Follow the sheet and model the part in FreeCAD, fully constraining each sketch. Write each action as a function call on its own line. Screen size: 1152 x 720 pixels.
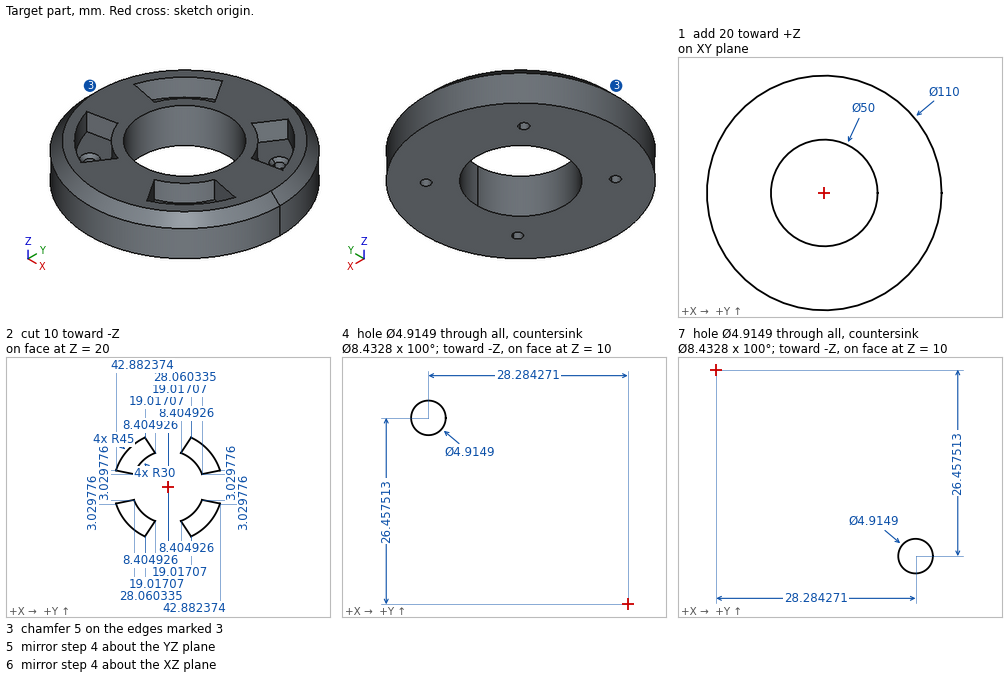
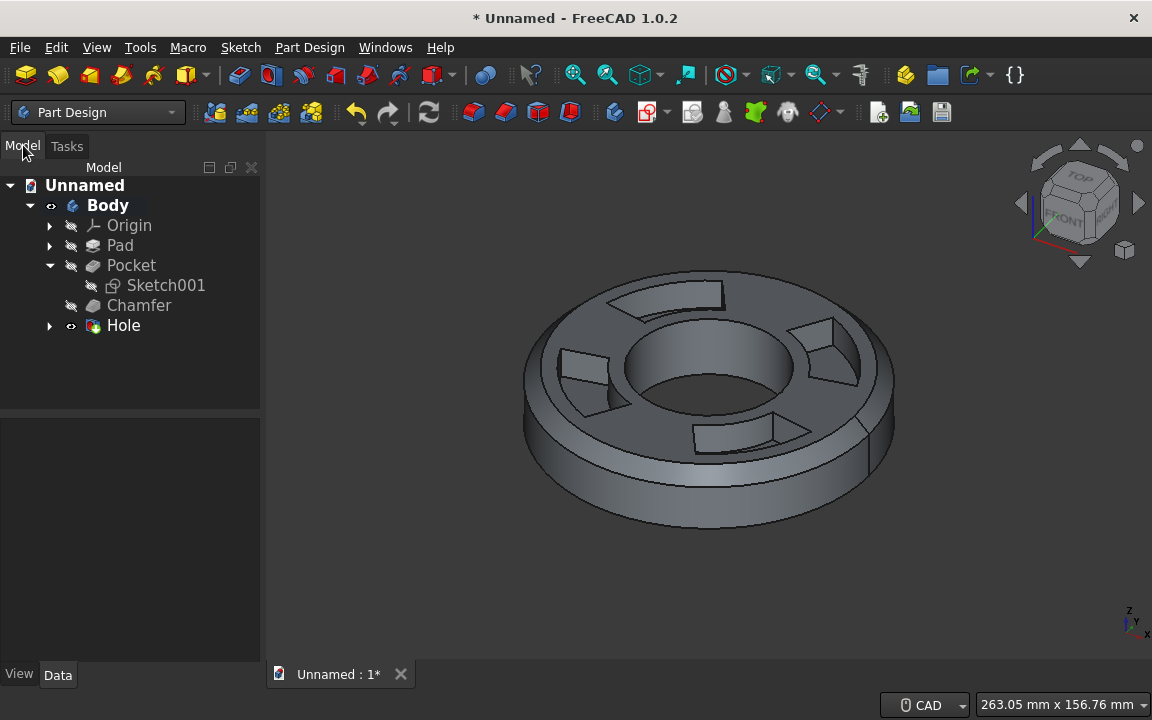
click(116, 326)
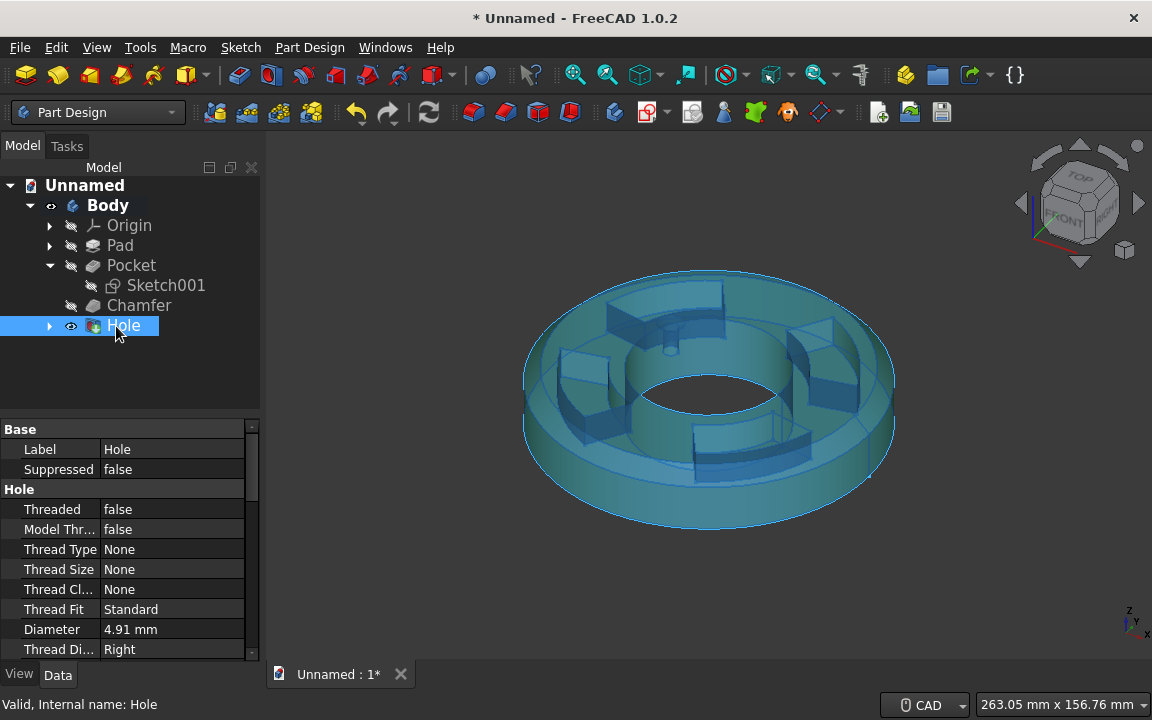
click(216, 112)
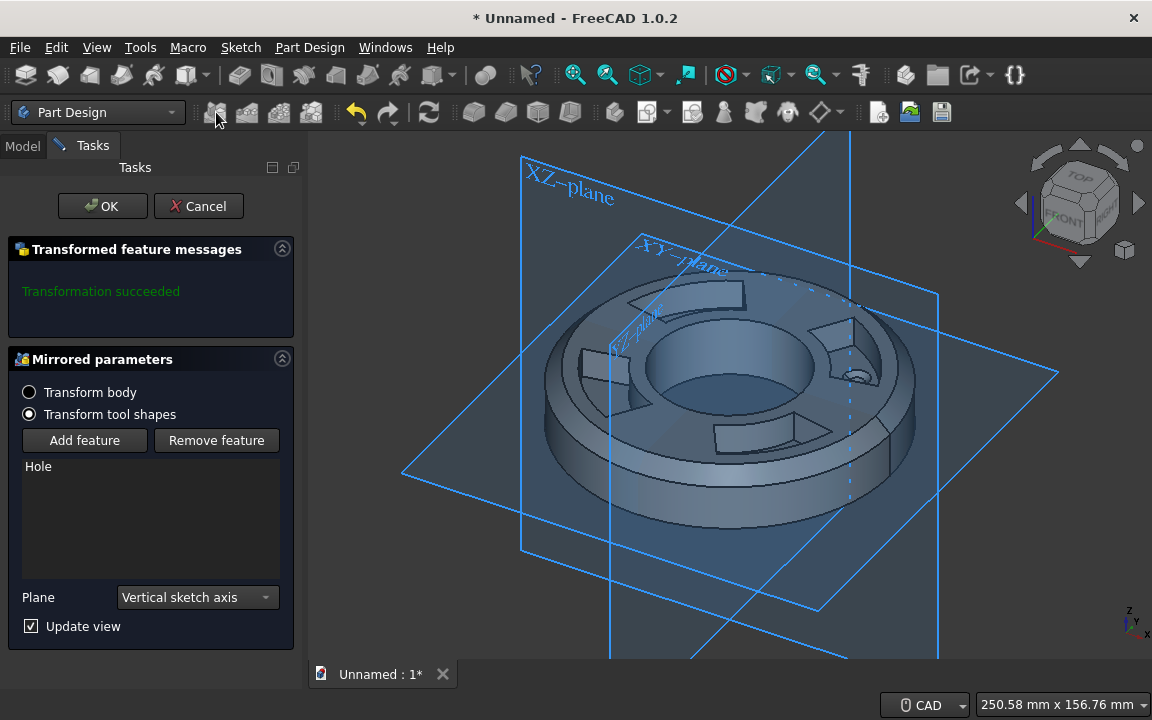
click(198, 598)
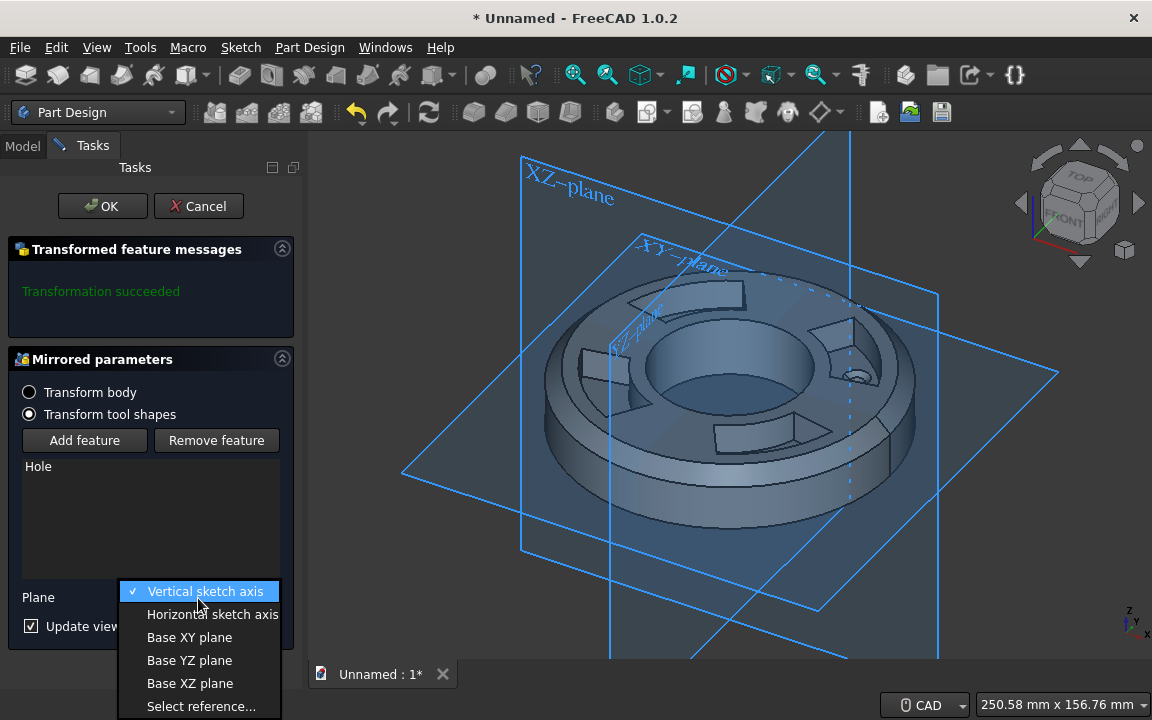
click(198, 660)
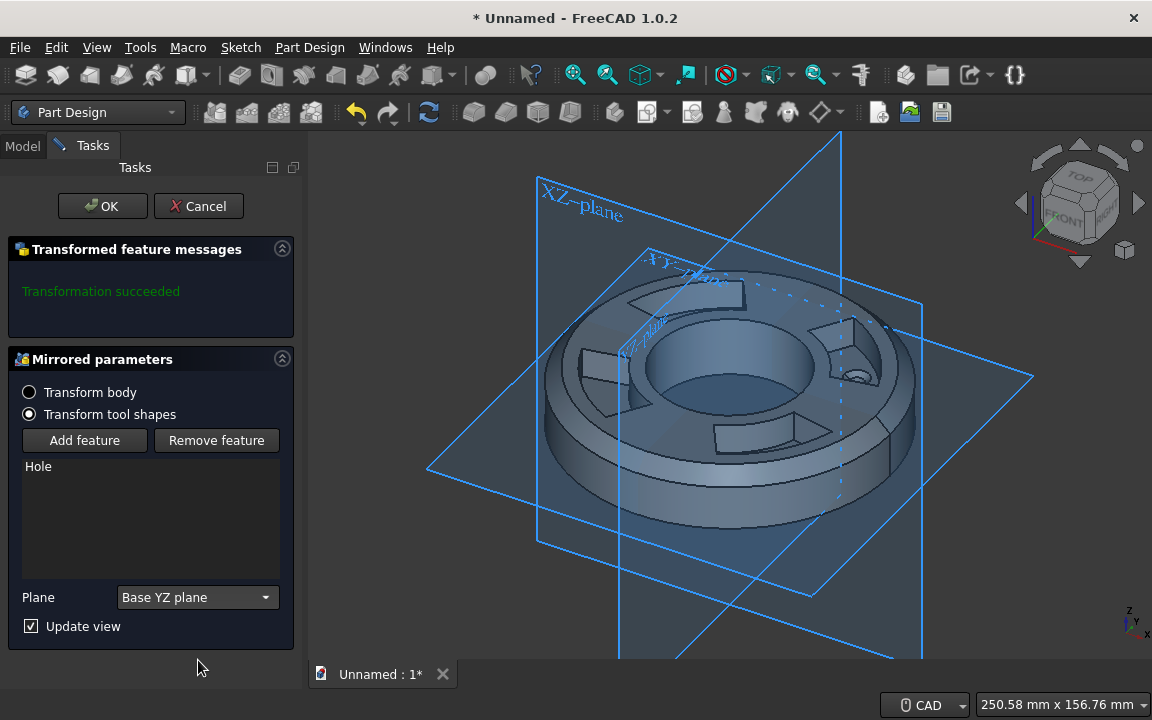
click(103, 206)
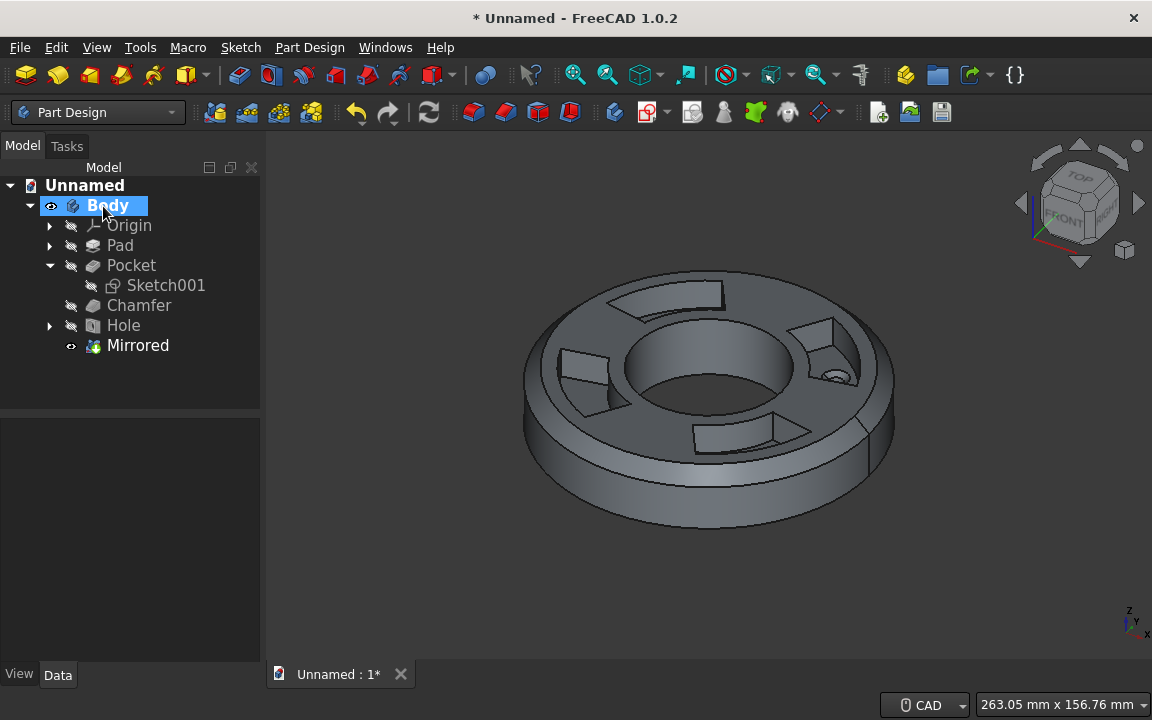
click(116, 326)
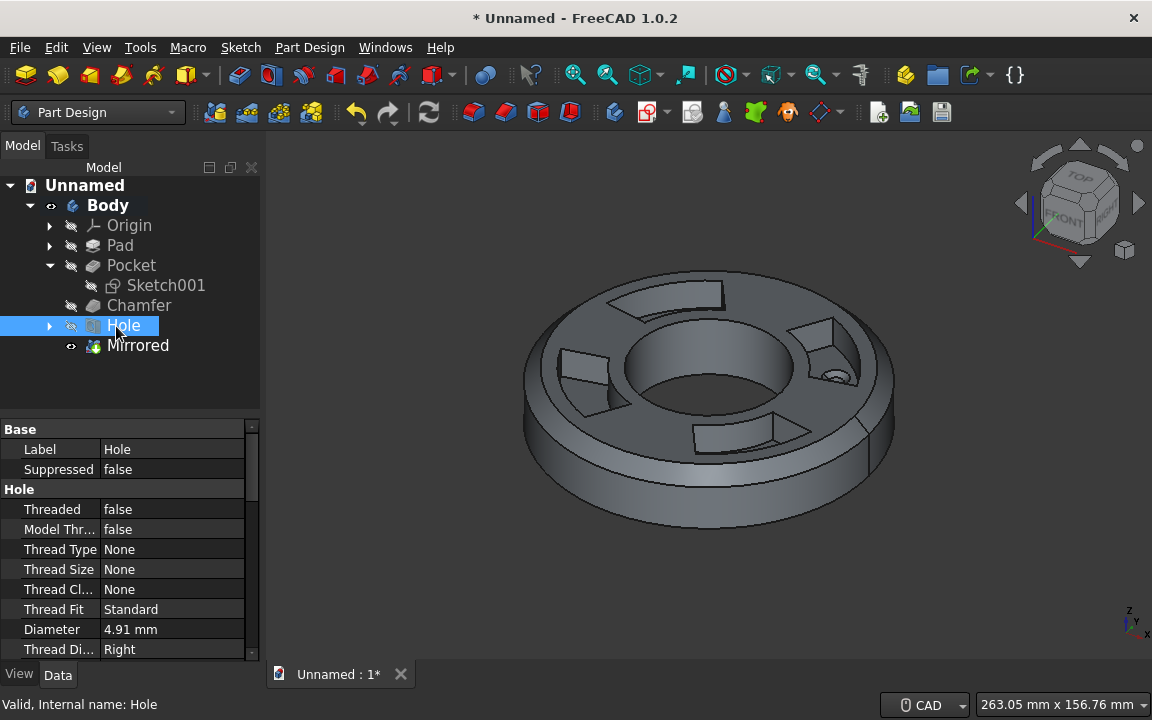
click(216, 112)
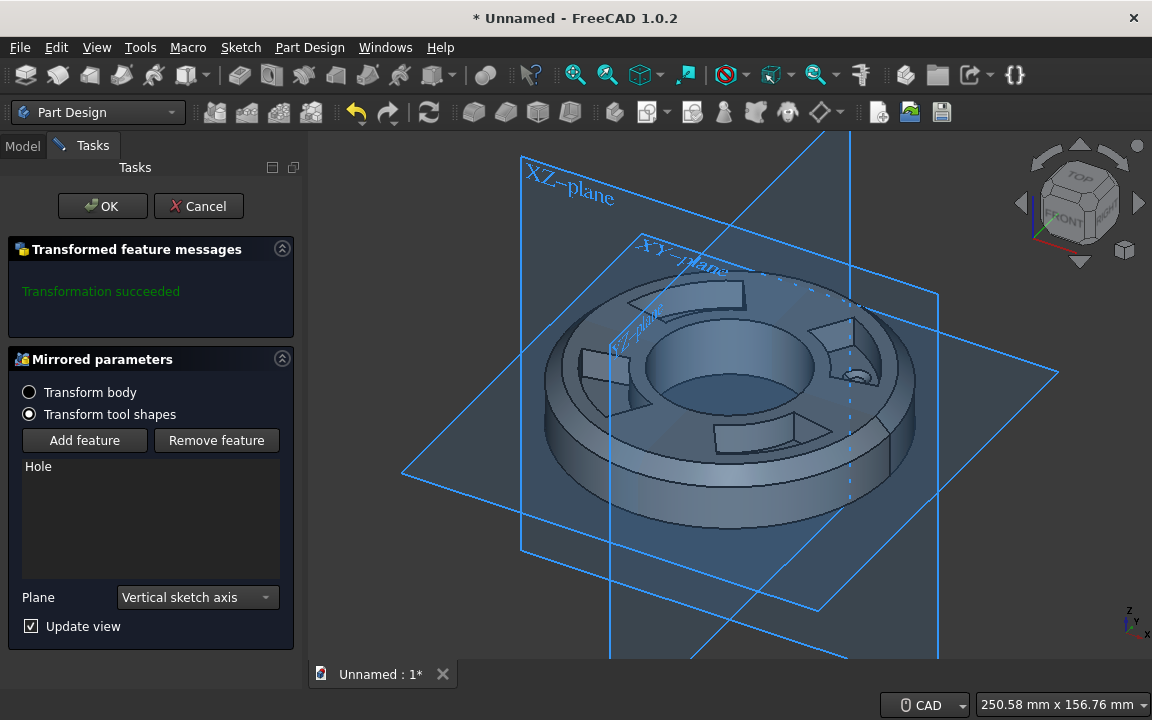
click(198, 598)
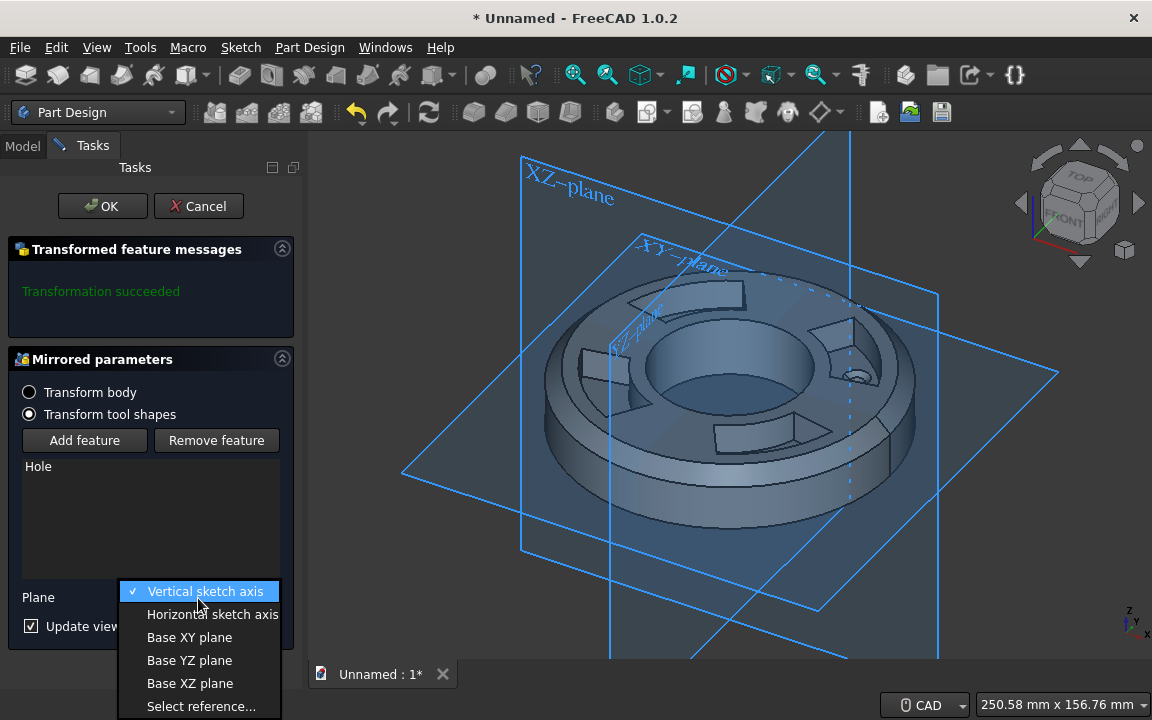
click(198, 684)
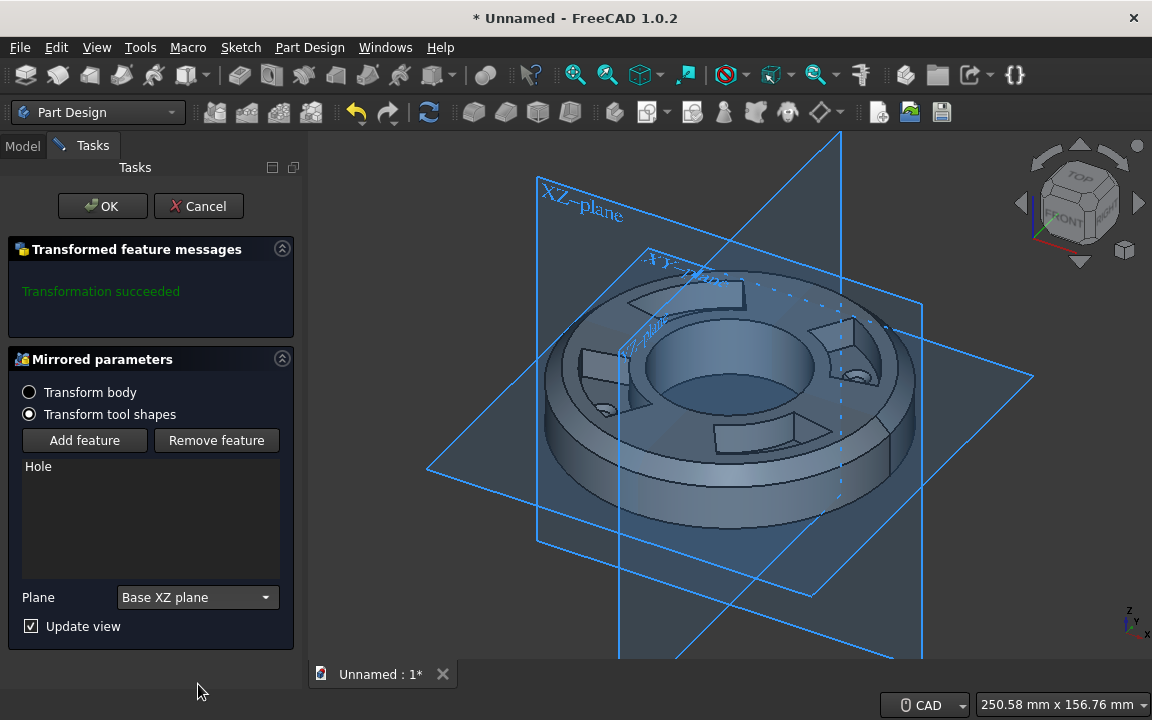
click(103, 206)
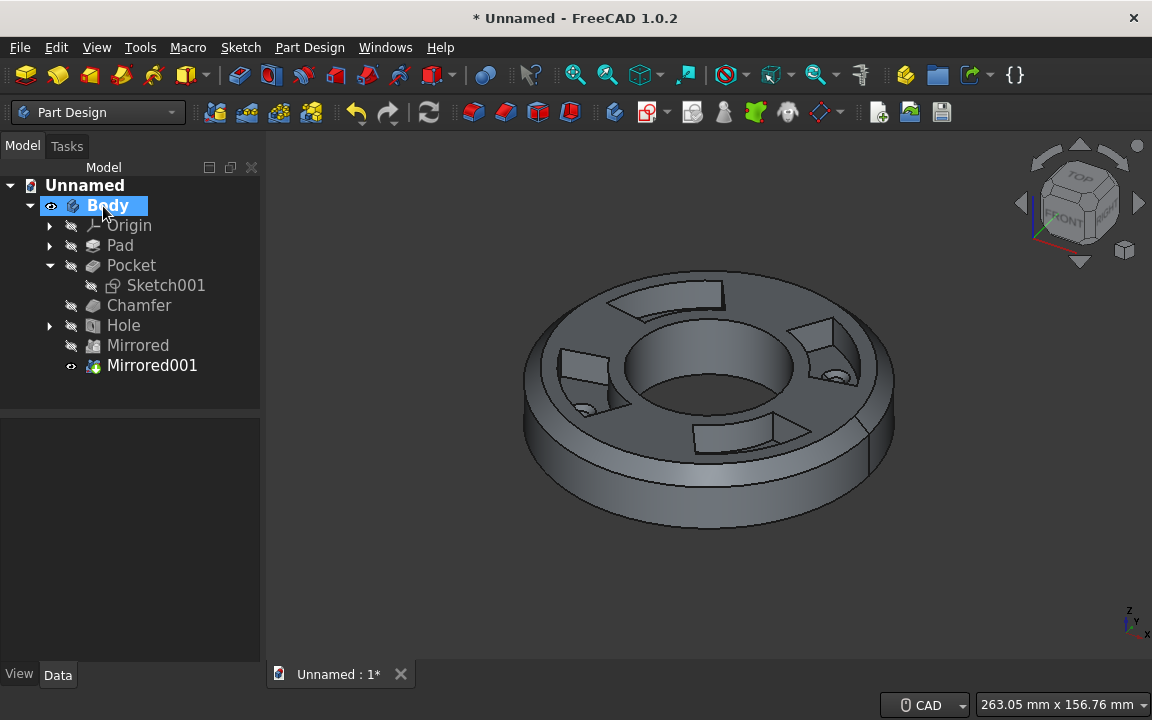
key(0)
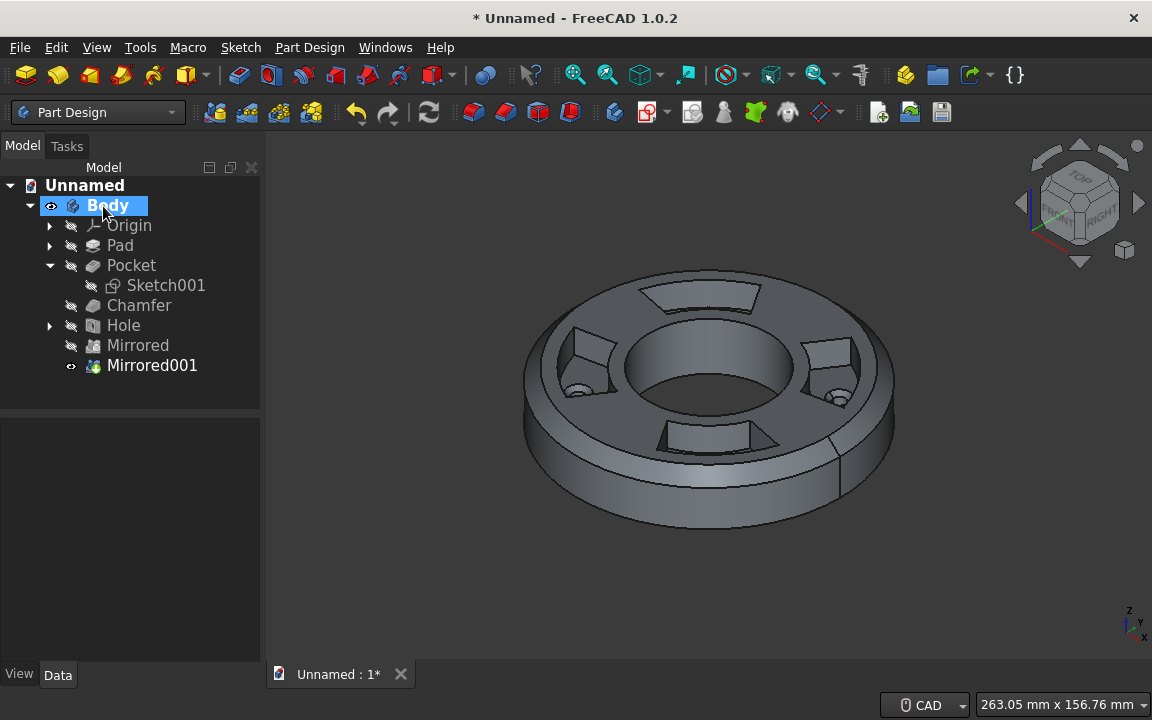
key(2)